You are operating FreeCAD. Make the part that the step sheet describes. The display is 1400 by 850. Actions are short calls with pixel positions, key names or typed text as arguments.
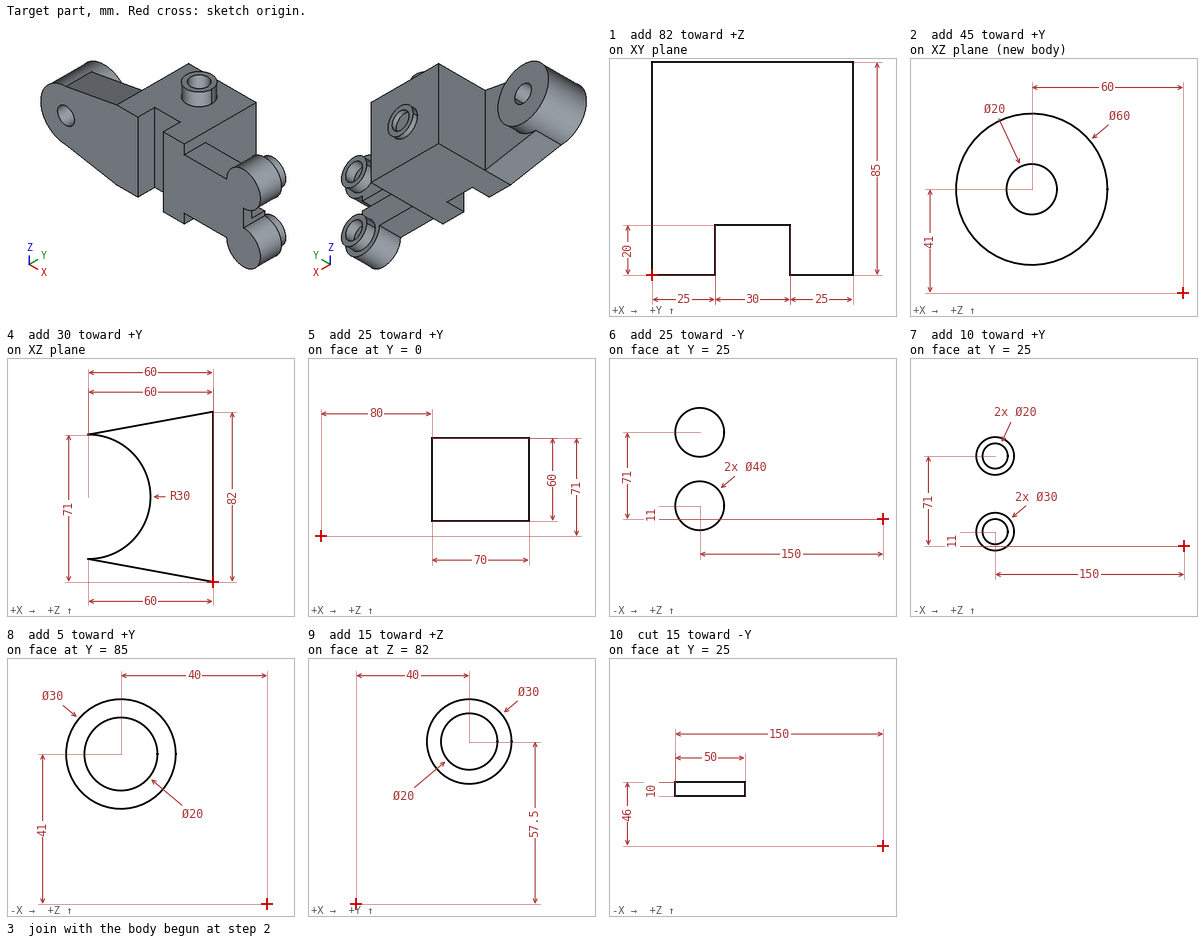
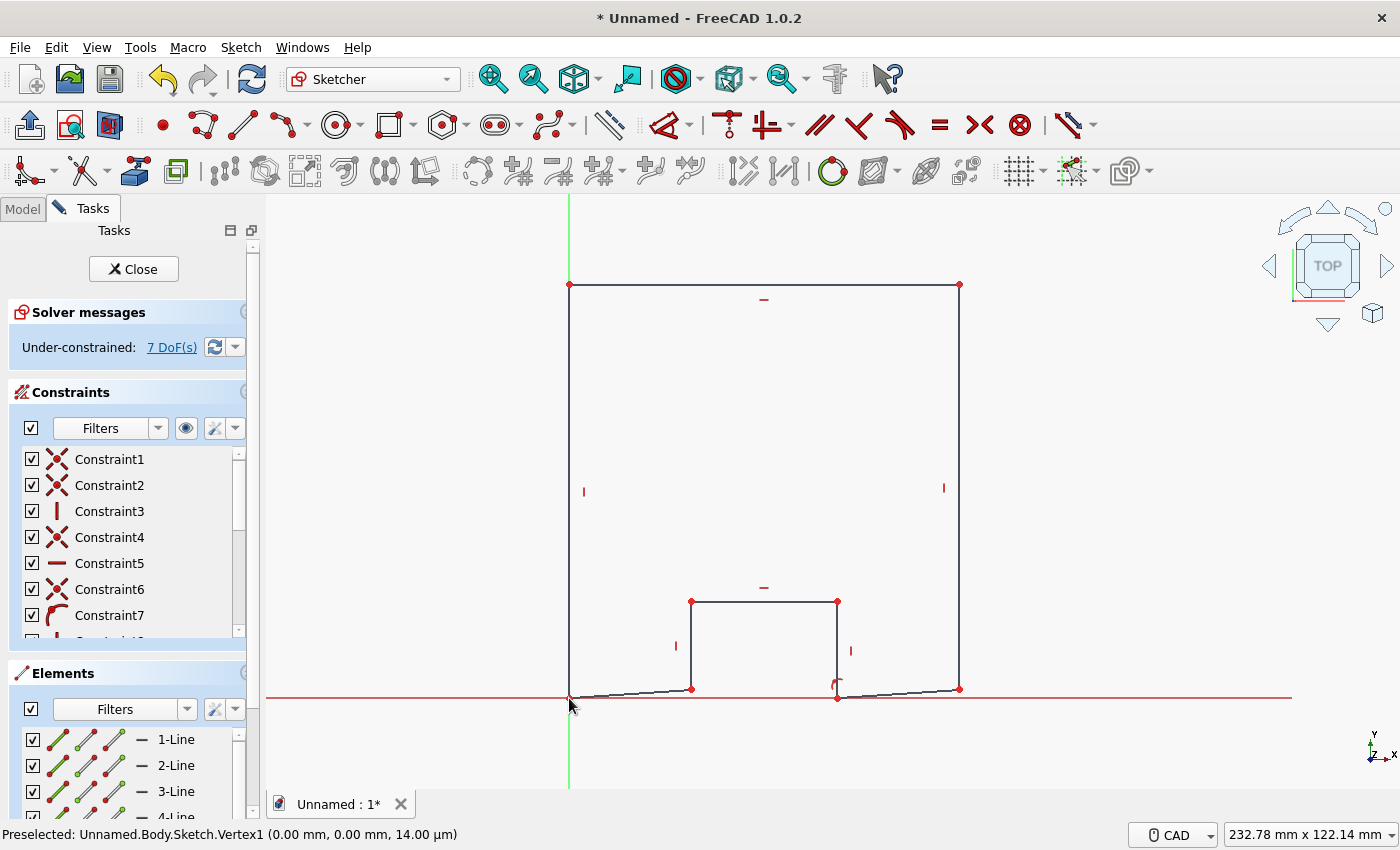
click(606, 696)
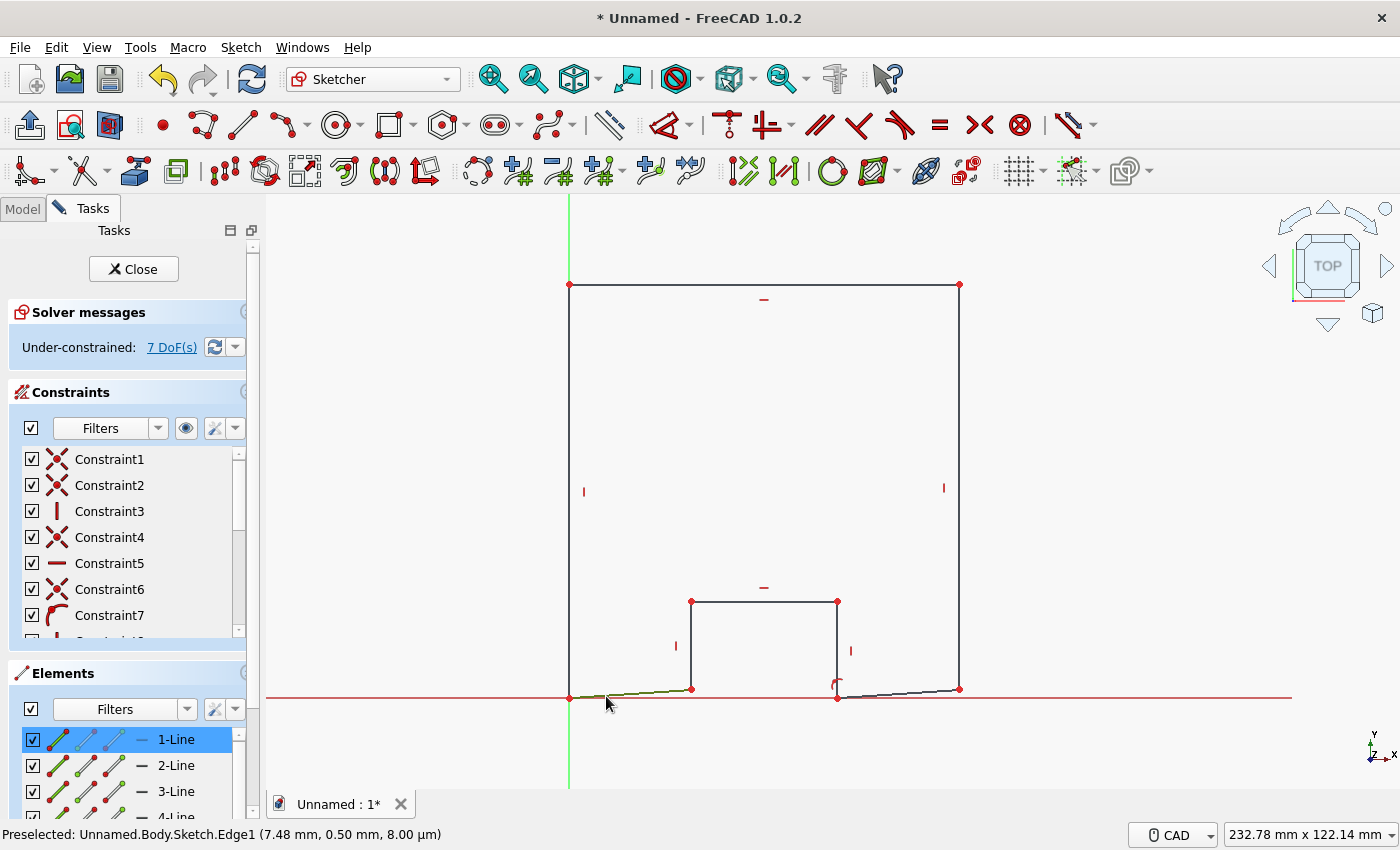
click(794, 126)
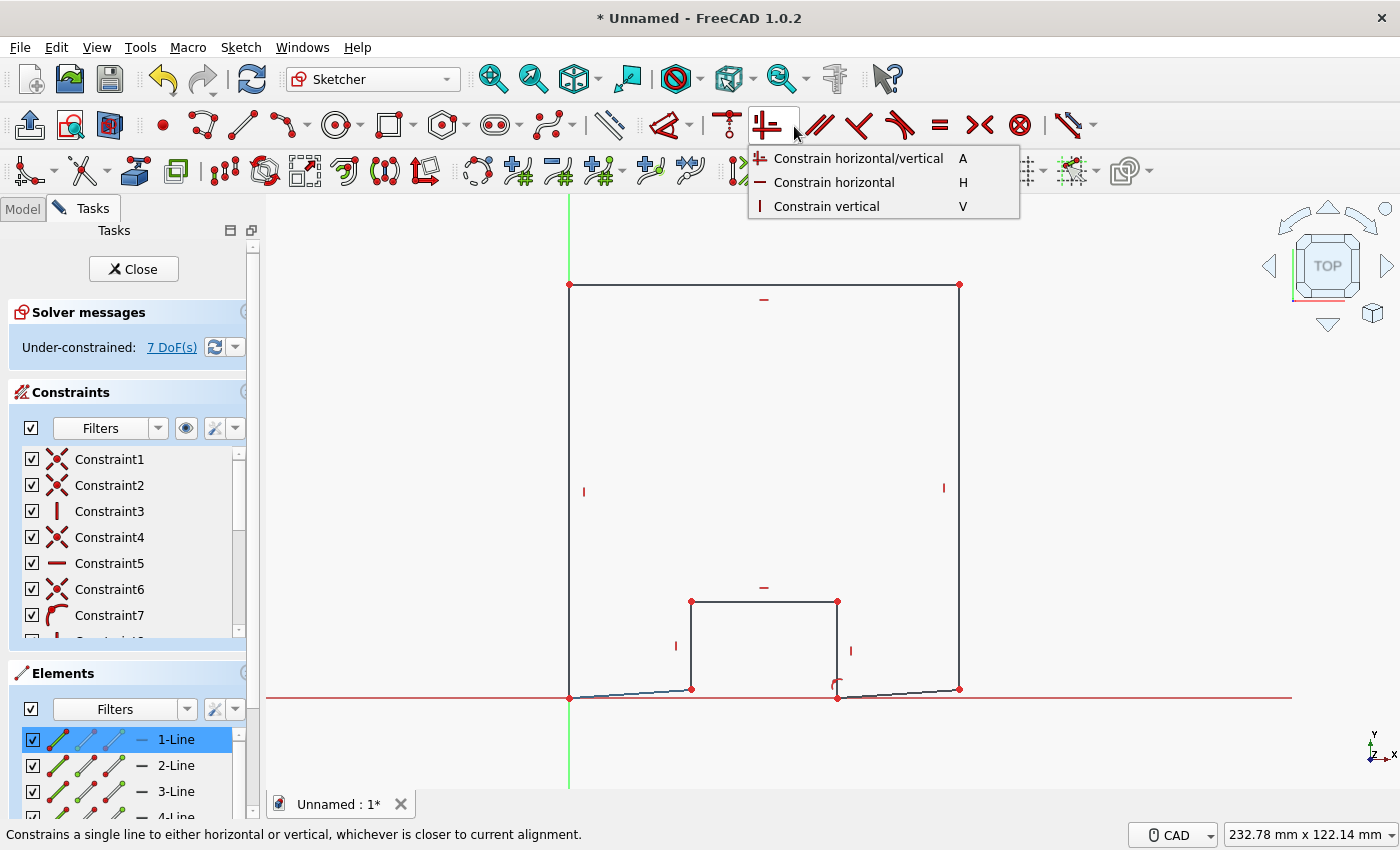
click(884, 182)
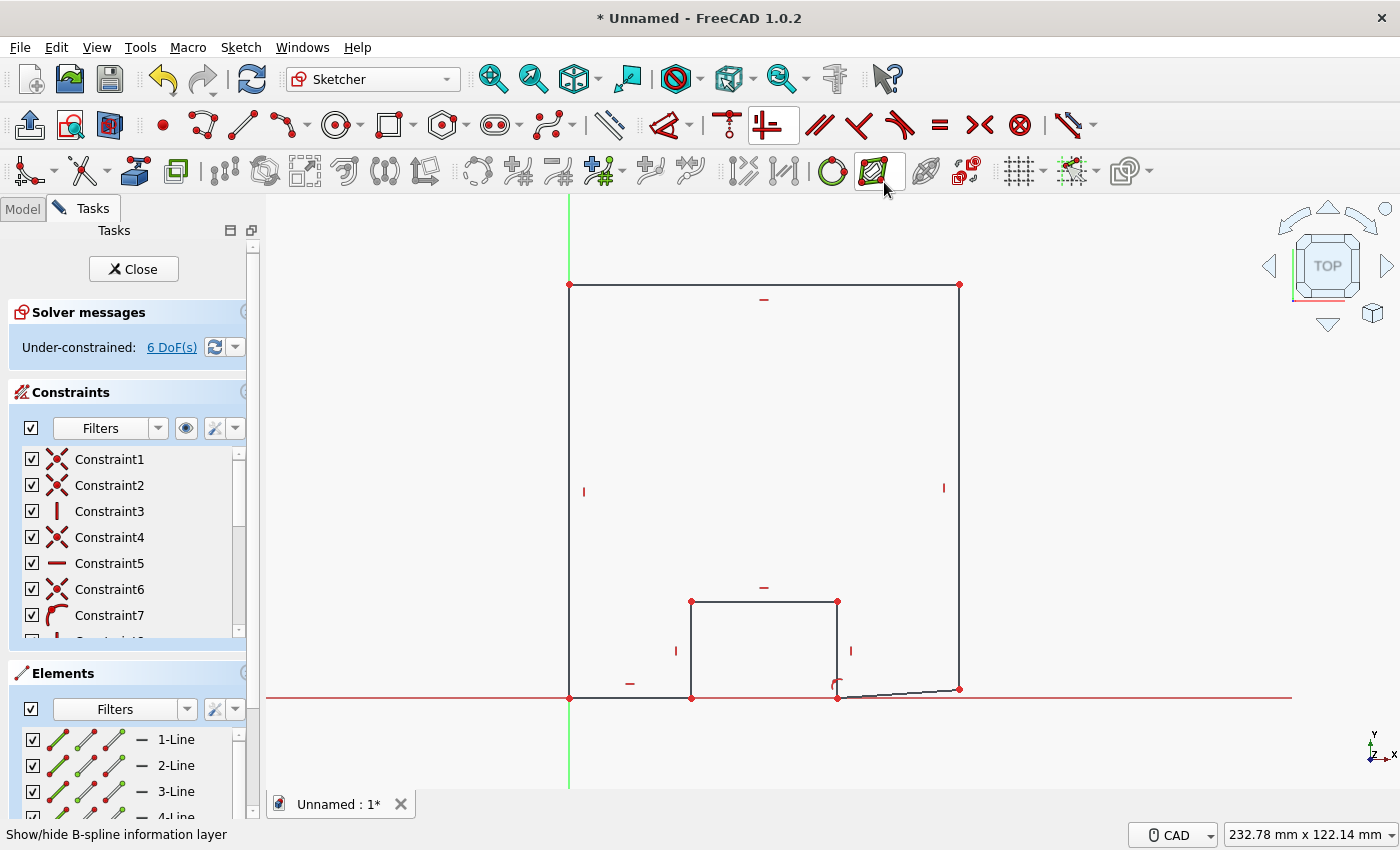
click(874, 696)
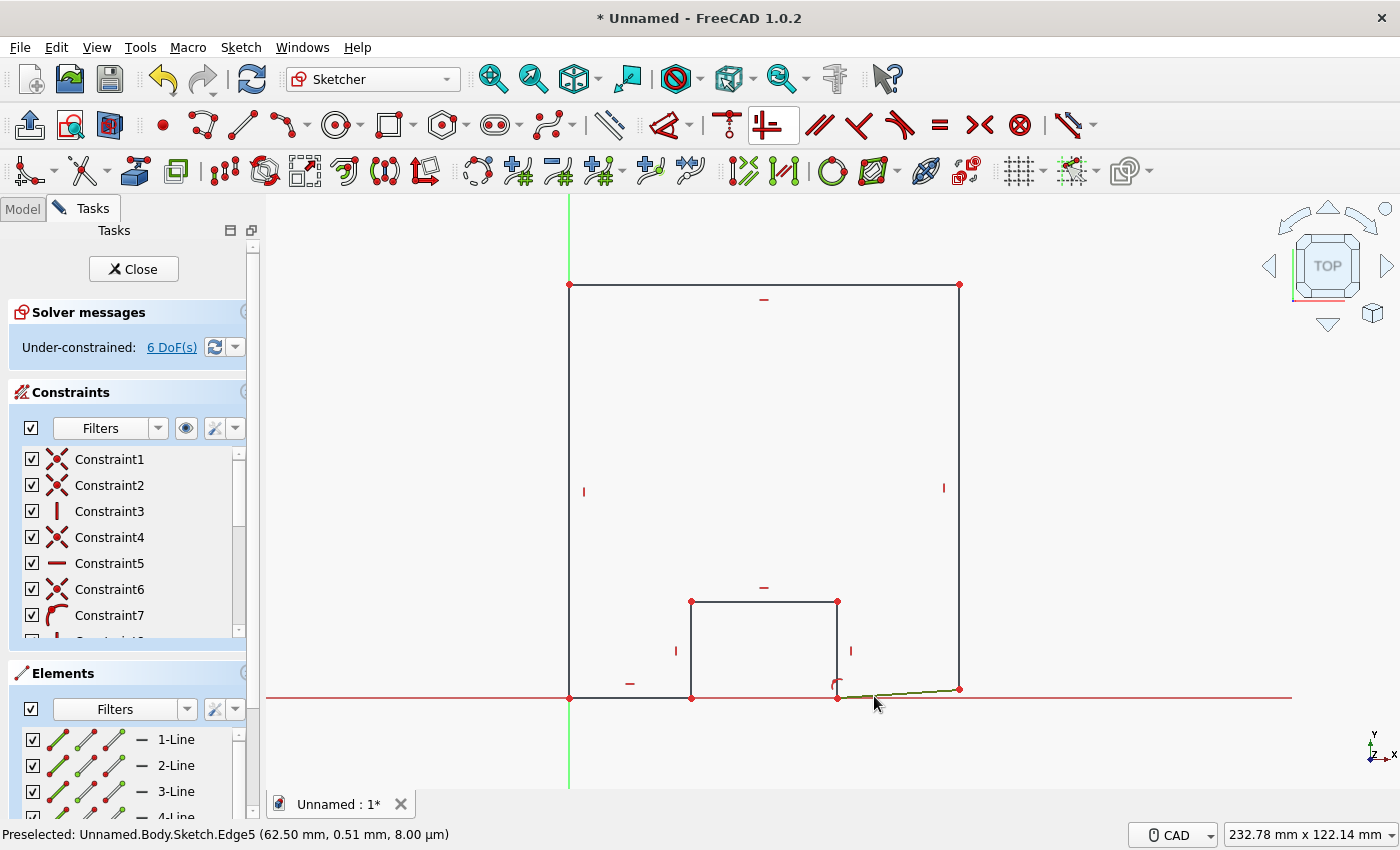
click(794, 126)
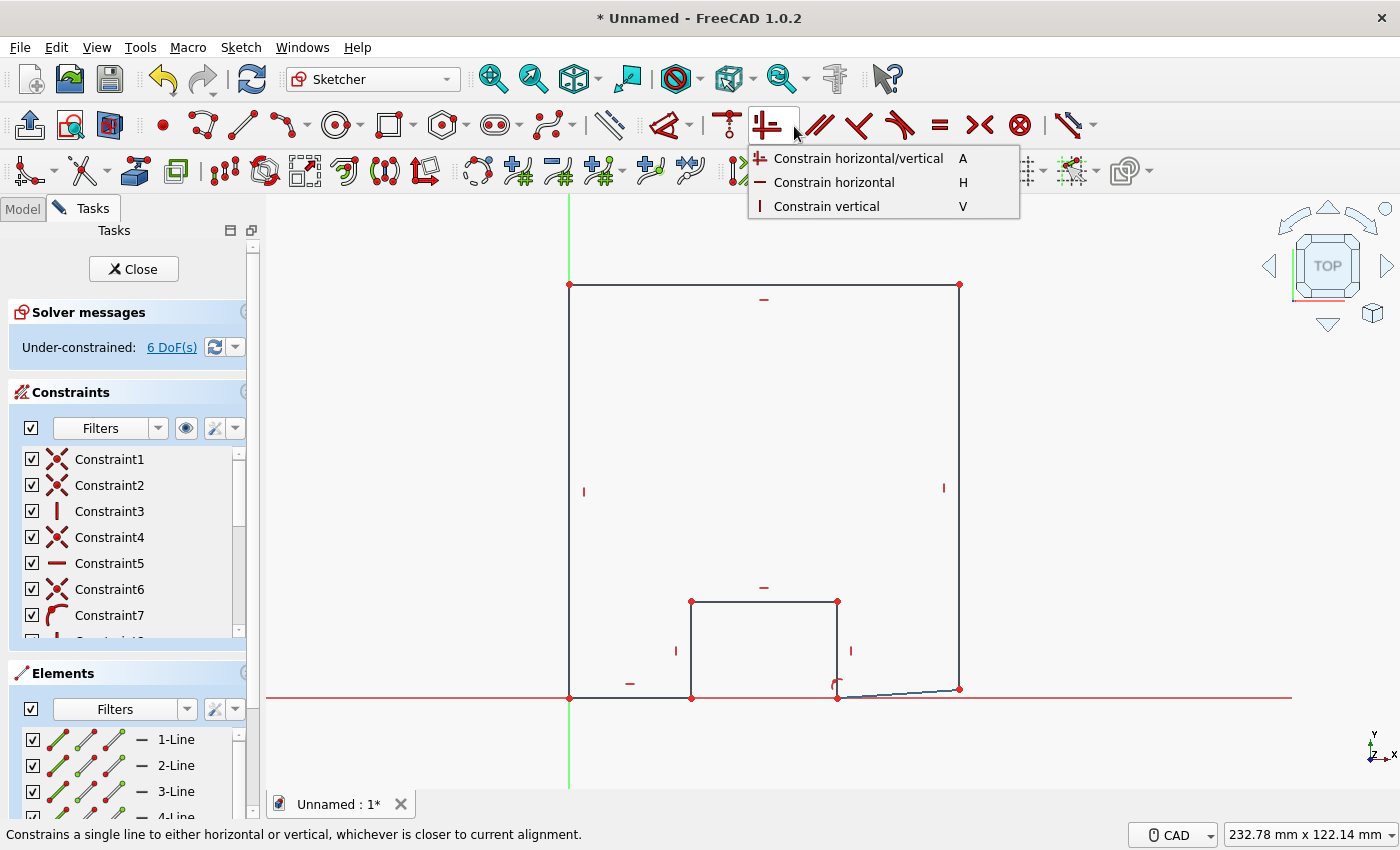
click(884, 182)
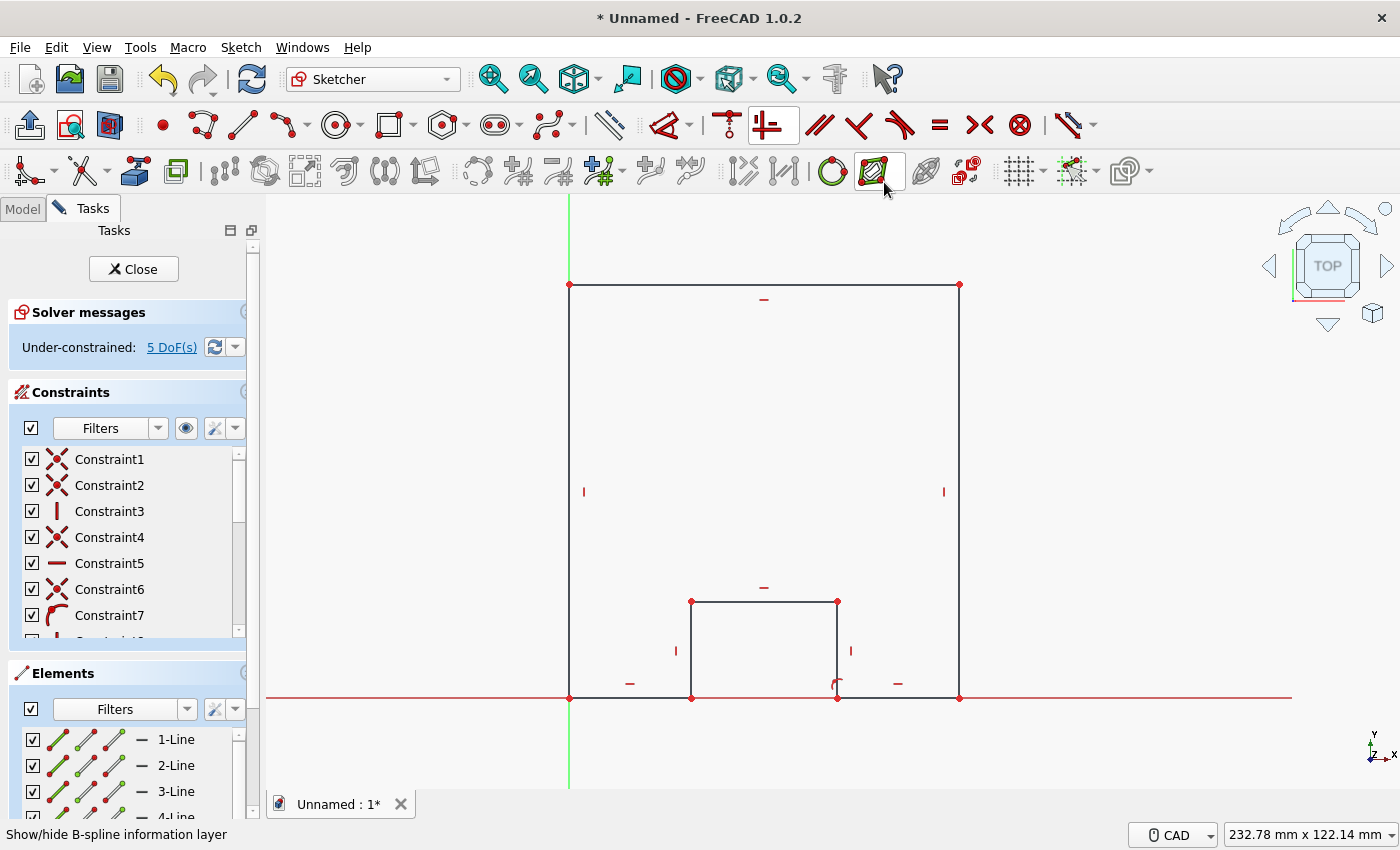
click(606, 698)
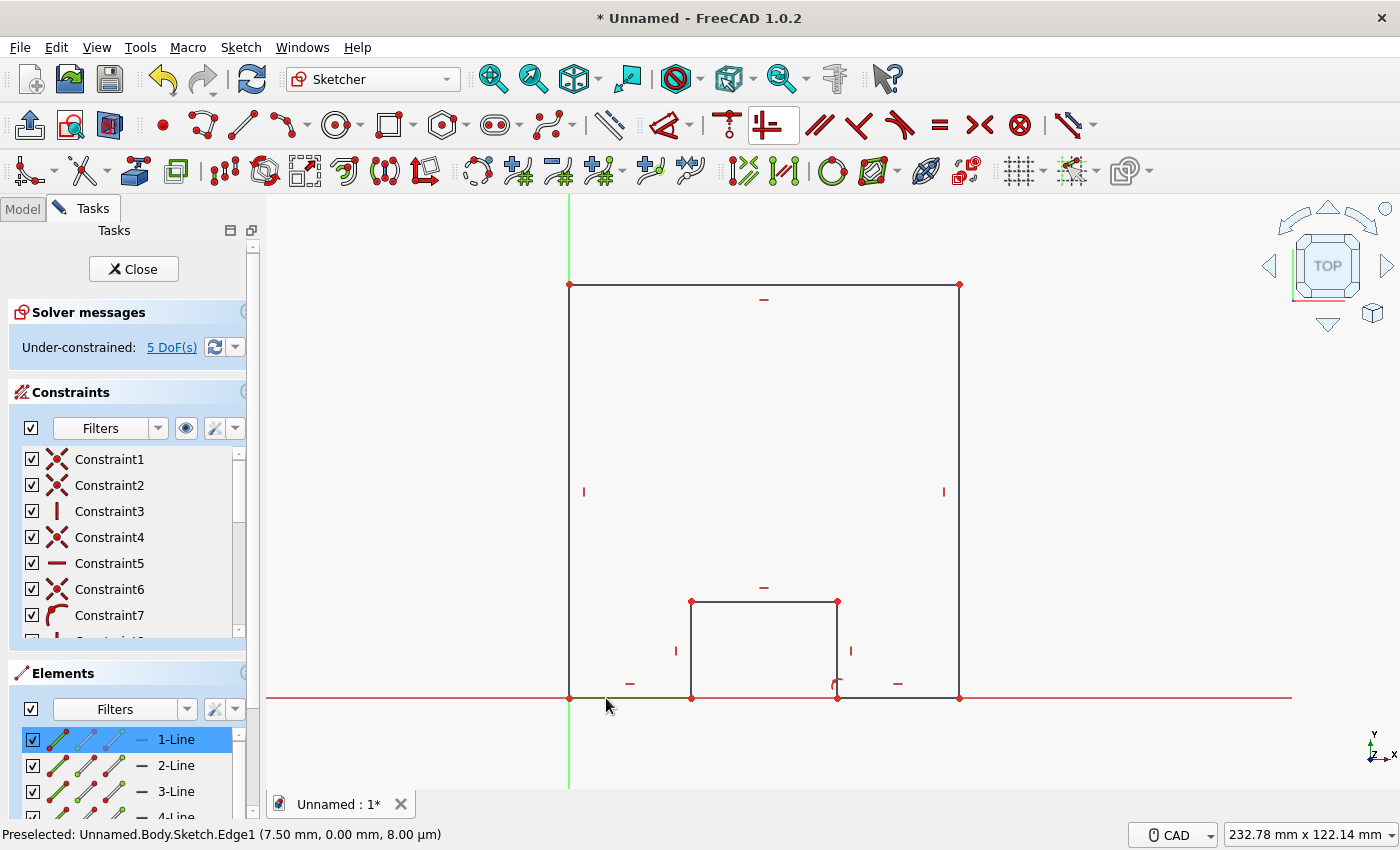
click(692, 126)